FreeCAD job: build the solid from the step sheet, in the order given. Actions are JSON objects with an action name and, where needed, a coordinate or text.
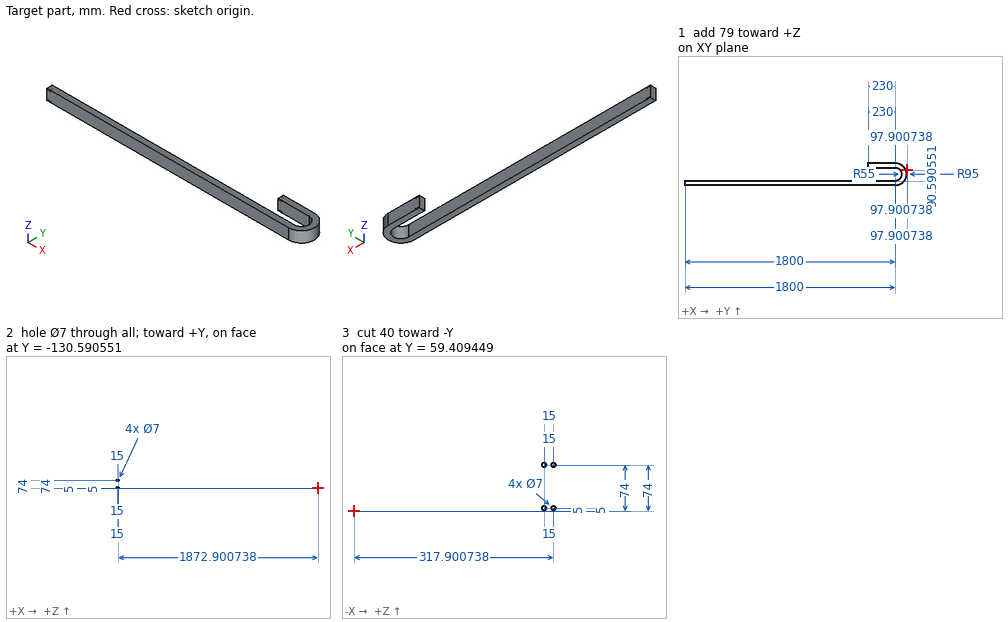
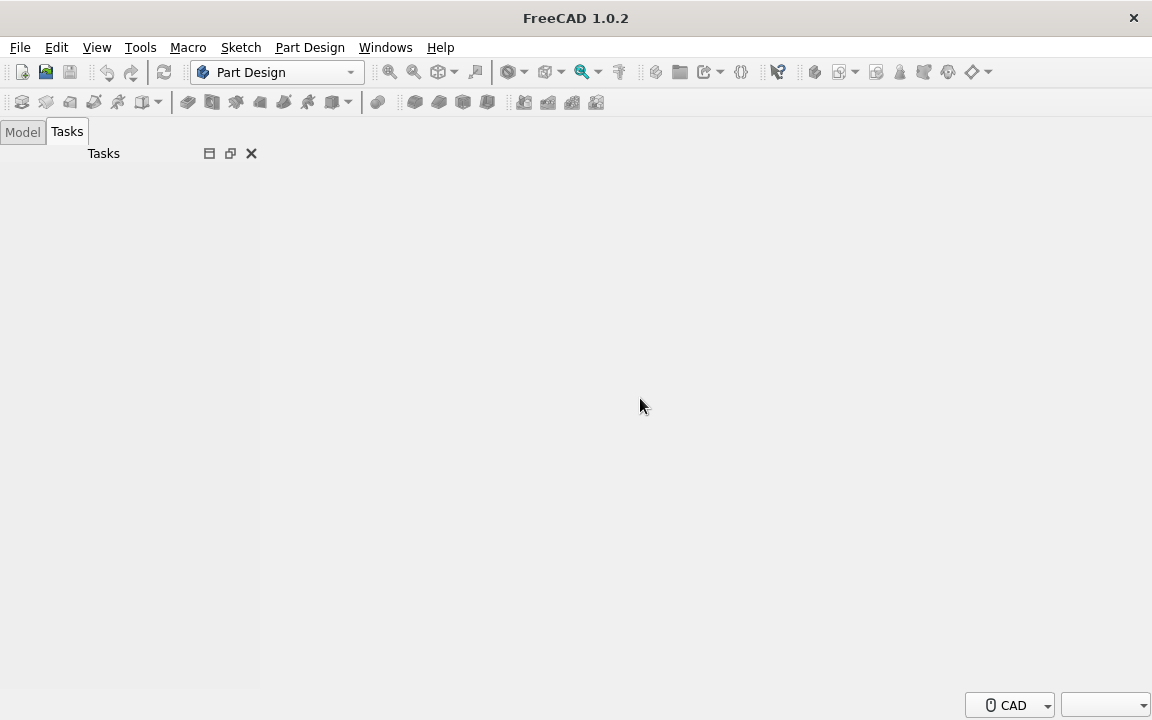
{"action": "key", "text": "ctrl+n"}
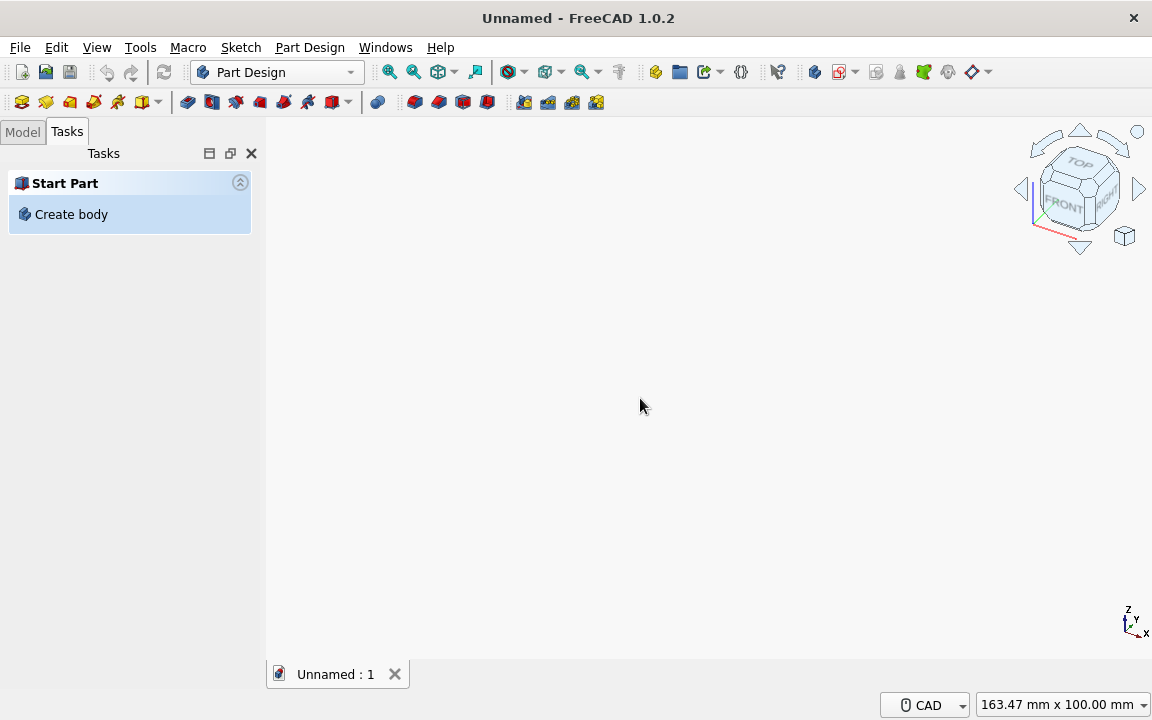
{"action": "left_click", "coordinate": [840, 72]}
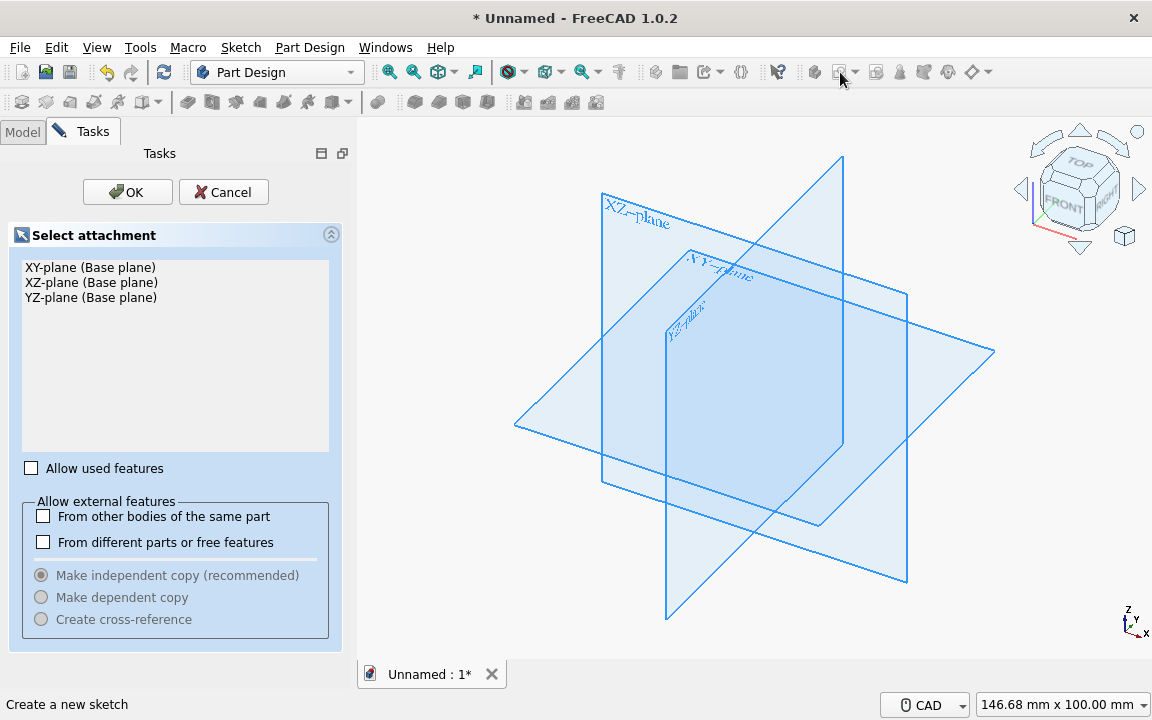
{"action": "left_click", "coordinate": [82, 268]}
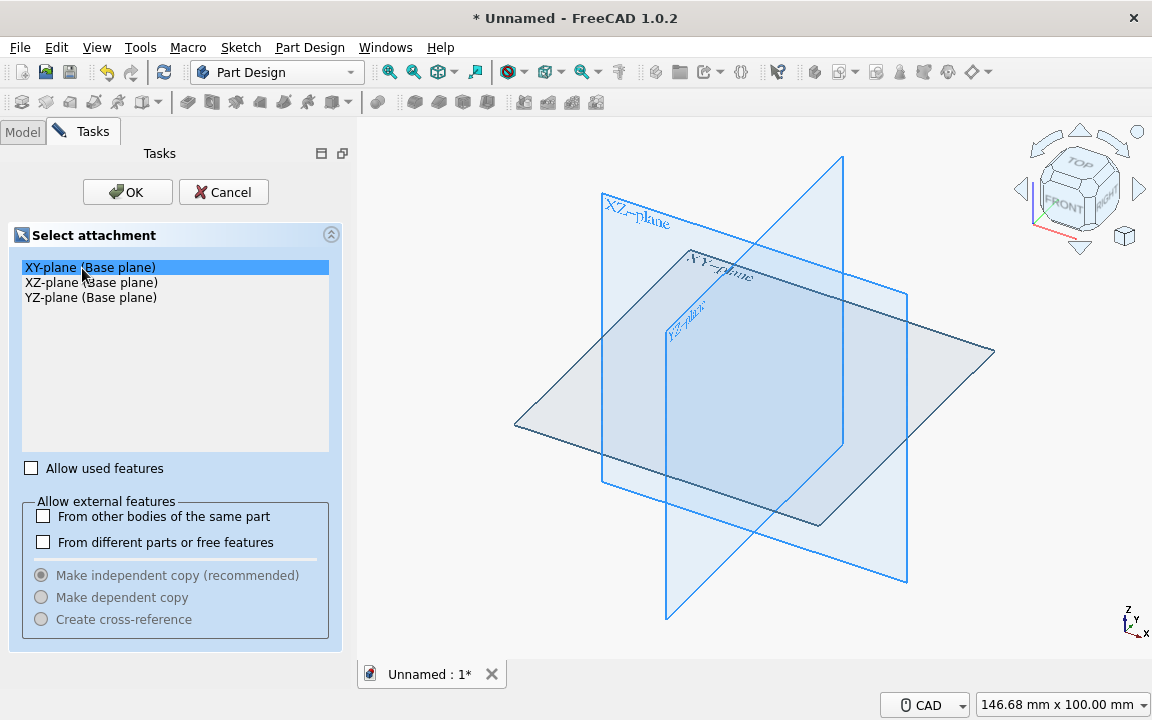
{"action": "left_click", "coordinate": [128, 192]}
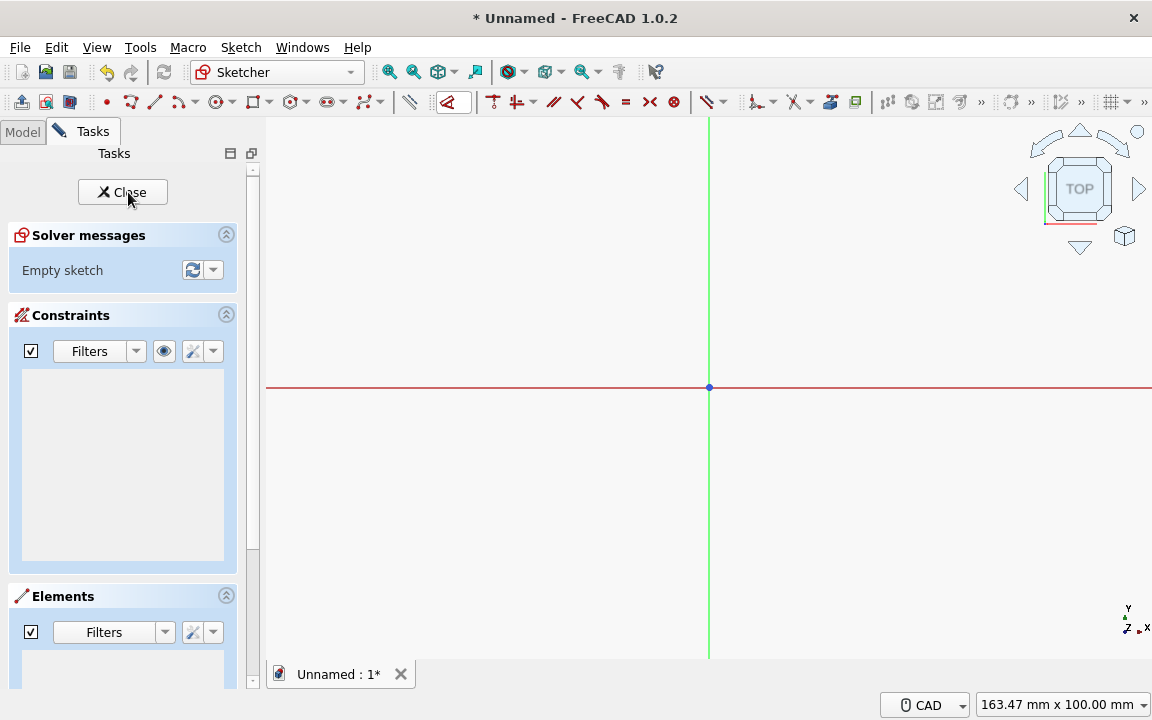
{"action": "scroll", "coordinate": [906, 378], "scroll_direction": "down", "scroll_amount": 15}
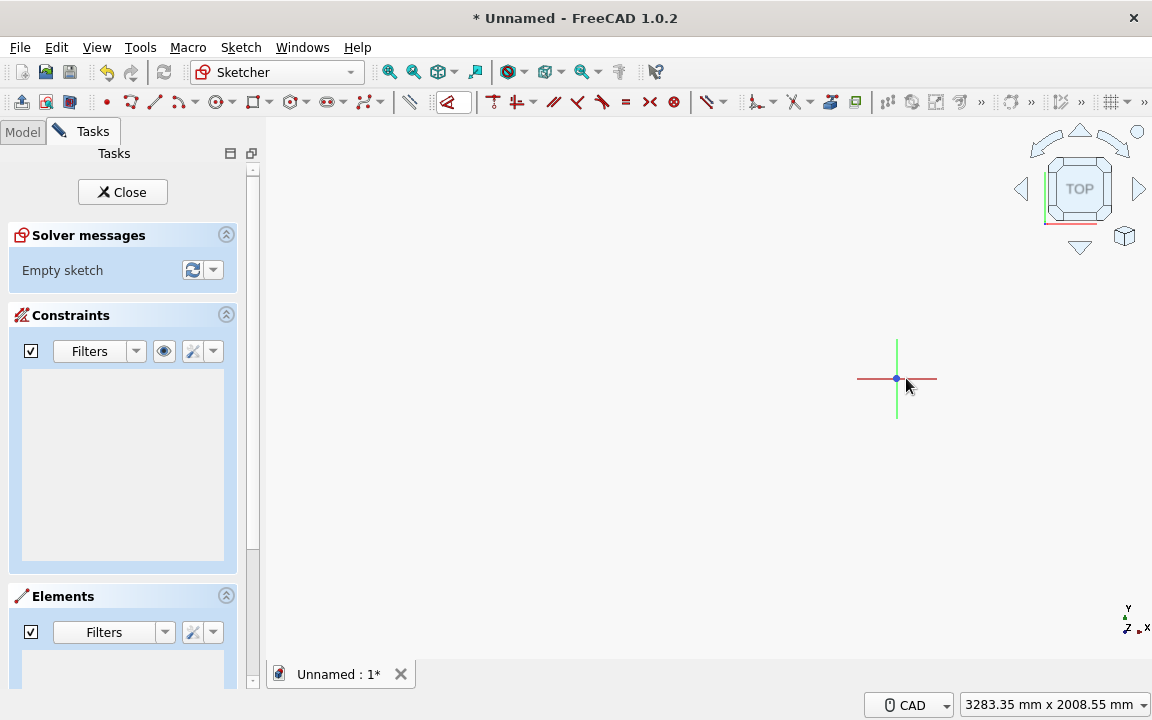
{"action": "key", "text": "g m"}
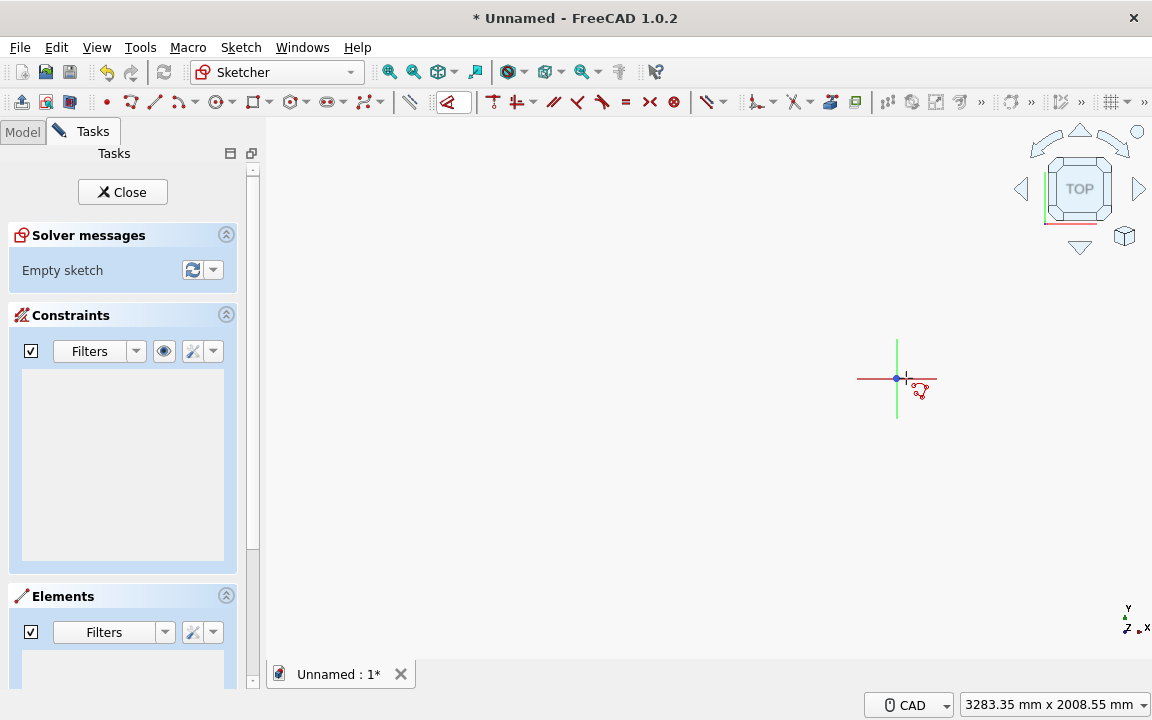
{"action": "left_click", "coordinate": [870, 403]}
{"action": "left_click", "coordinate": [385, 403]}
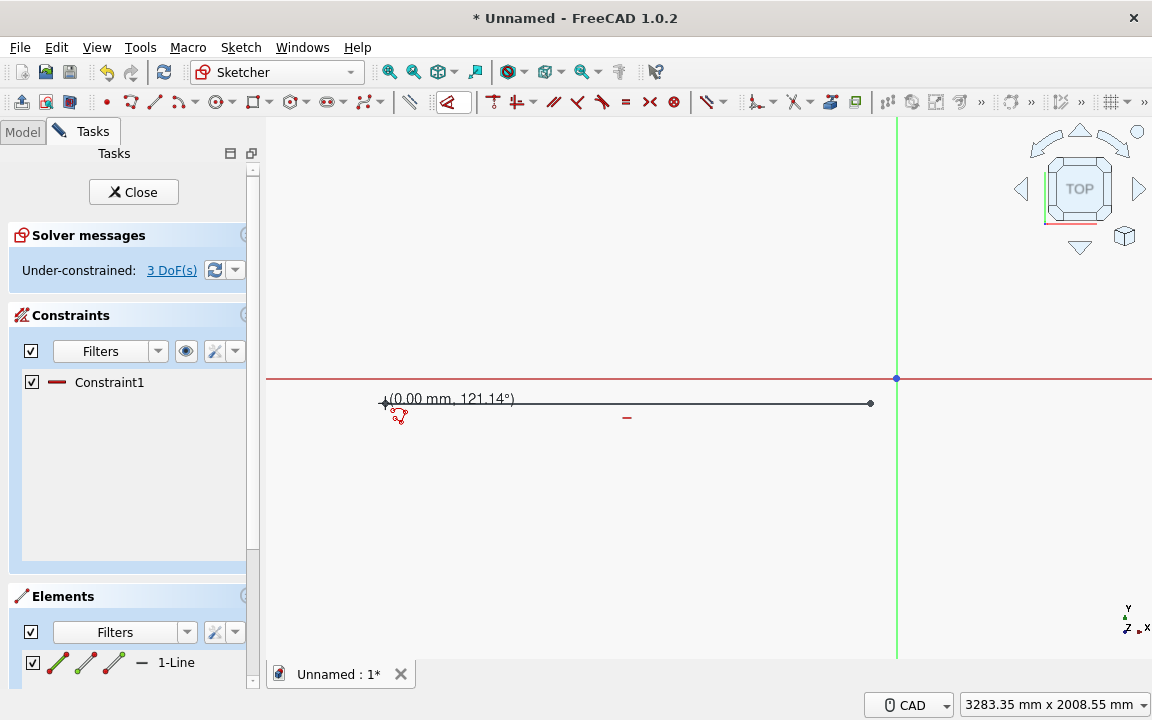
{"action": "scroll", "coordinate": [385, 414], "scroll_direction": "up", "scroll_amount": 2}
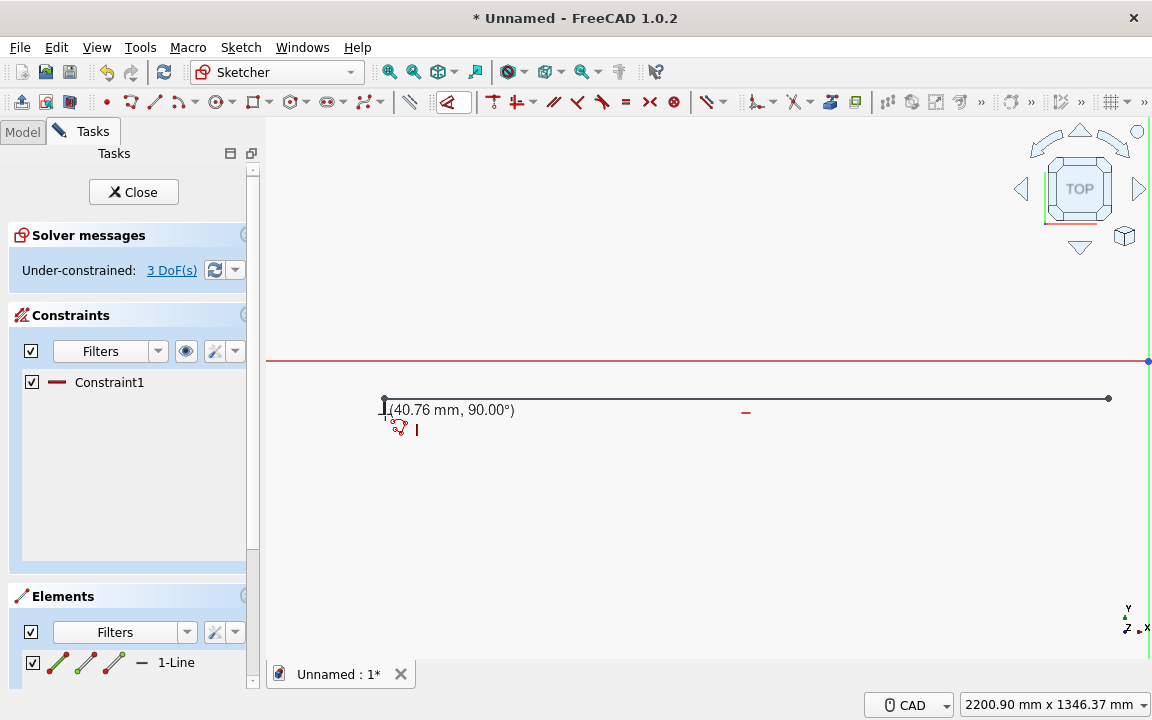
{"action": "left_click", "coordinate": [385, 414]}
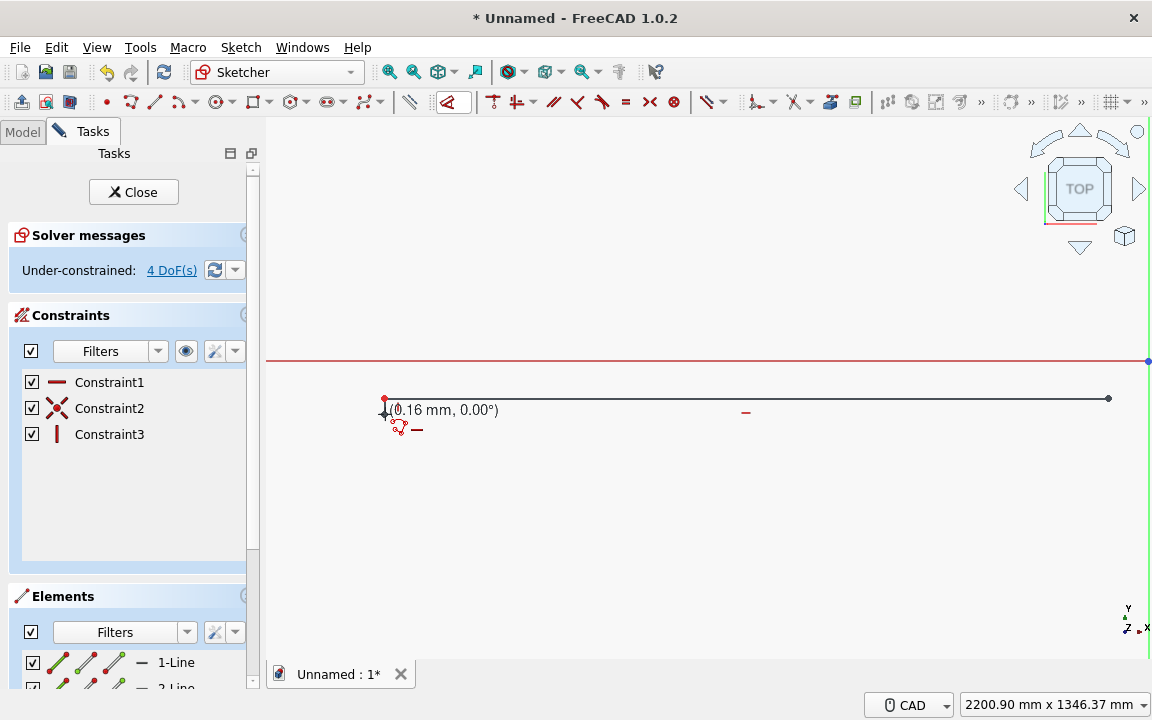
{"action": "scroll", "coordinate": [384, 413], "scroll_direction": "down", "scroll_amount": 2}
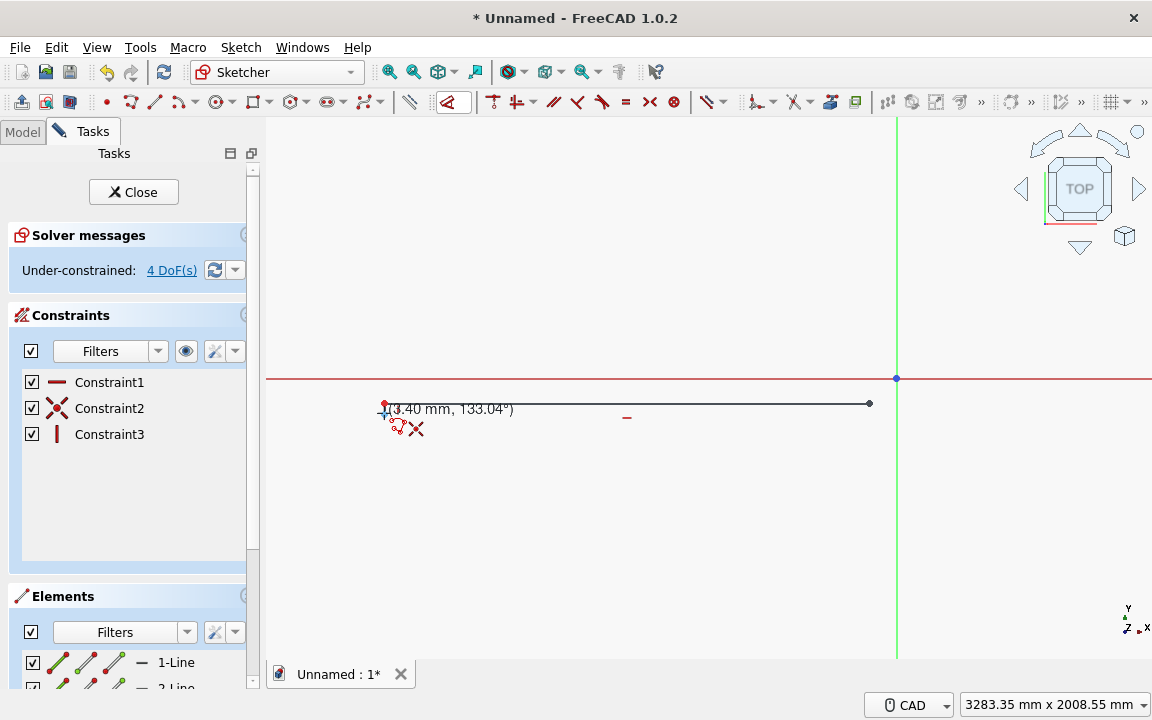
{"action": "scroll", "coordinate": [870, 414], "scroll_direction": "up", "scroll_amount": 2}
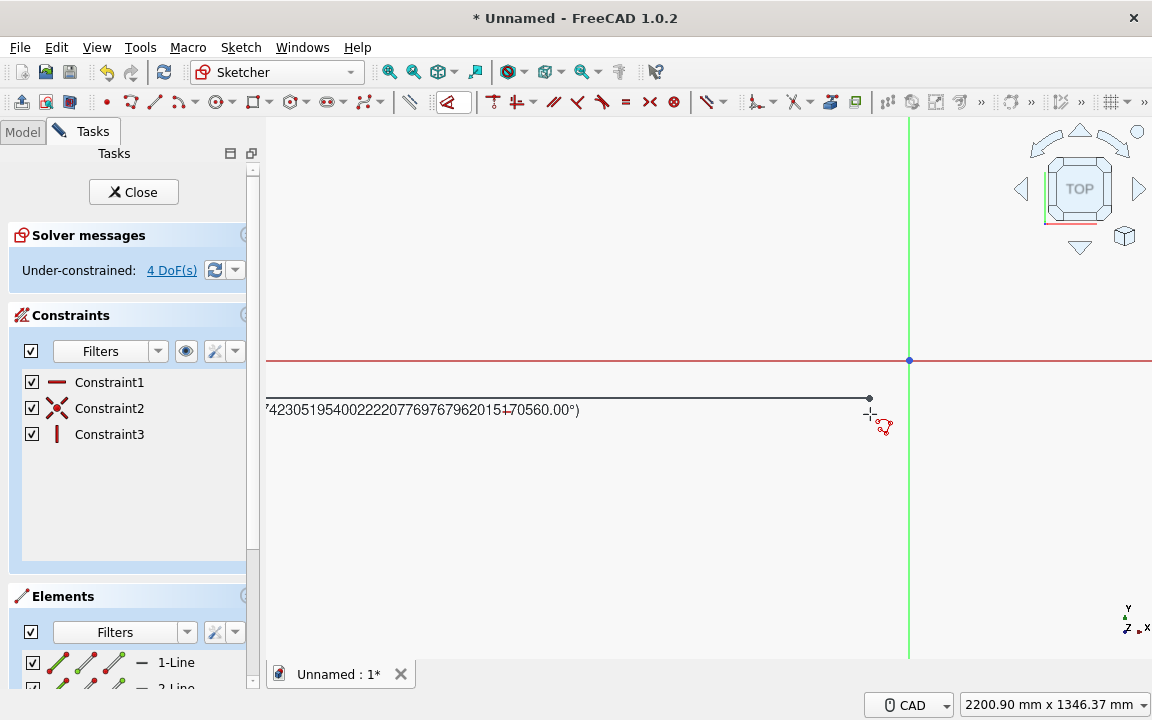
{"action": "left_click", "coordinate": [870, 414]}
{"action": "right_click", "coordinate": [870, 414]}